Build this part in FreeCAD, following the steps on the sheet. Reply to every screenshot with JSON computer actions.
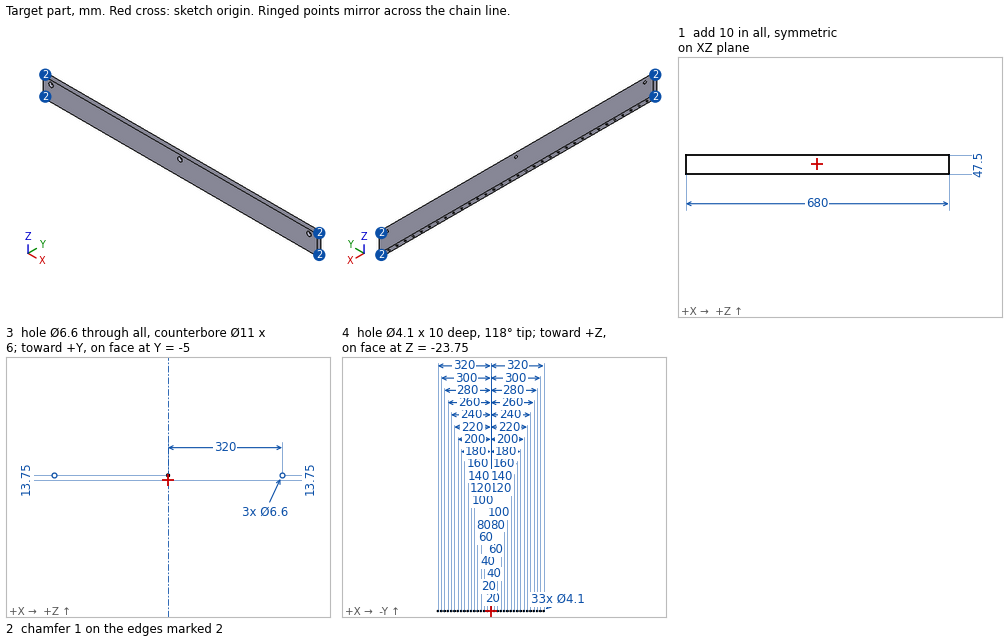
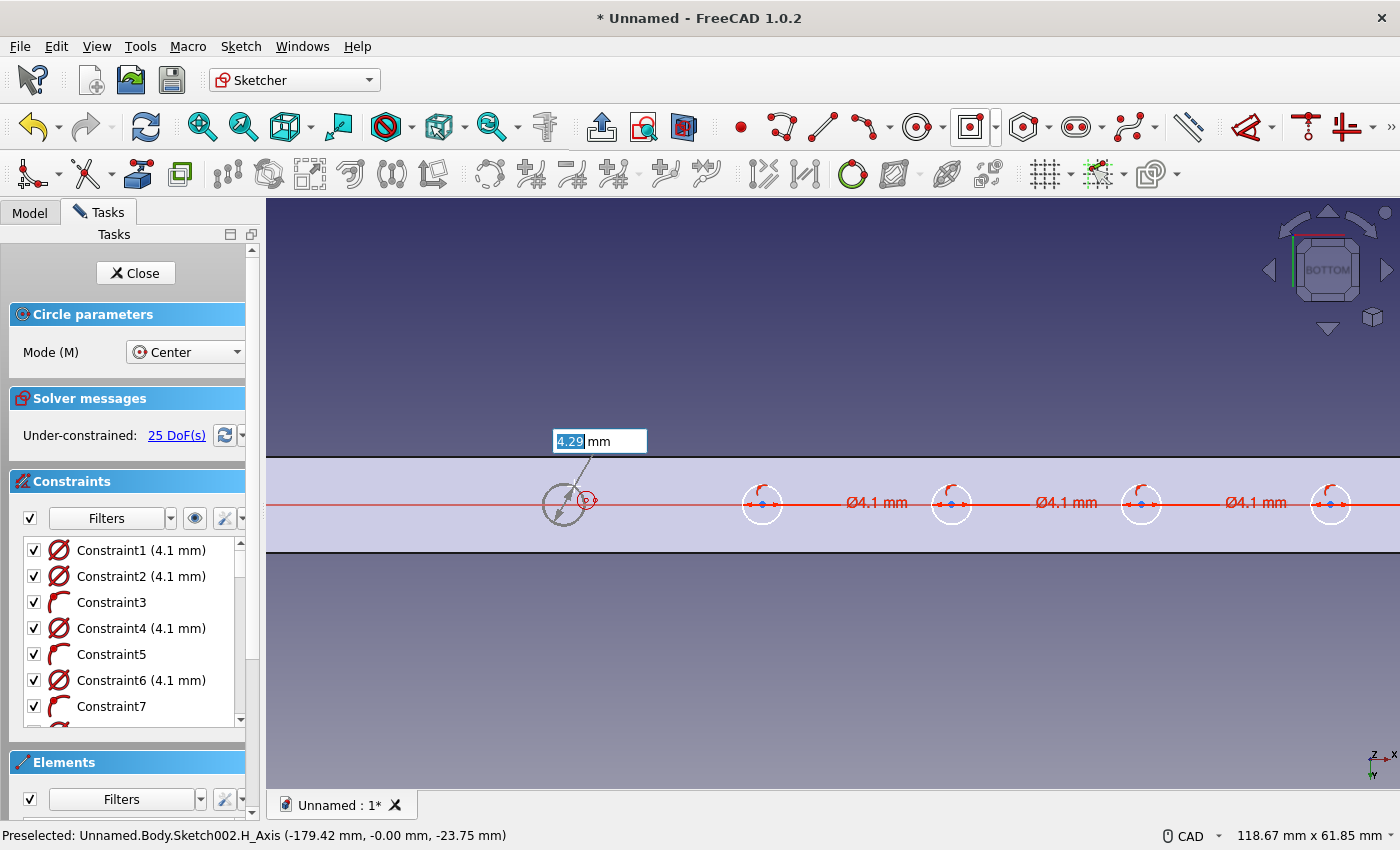
{"action": "type", "text": "4.1"}
{"action": "key", "text": "Return"}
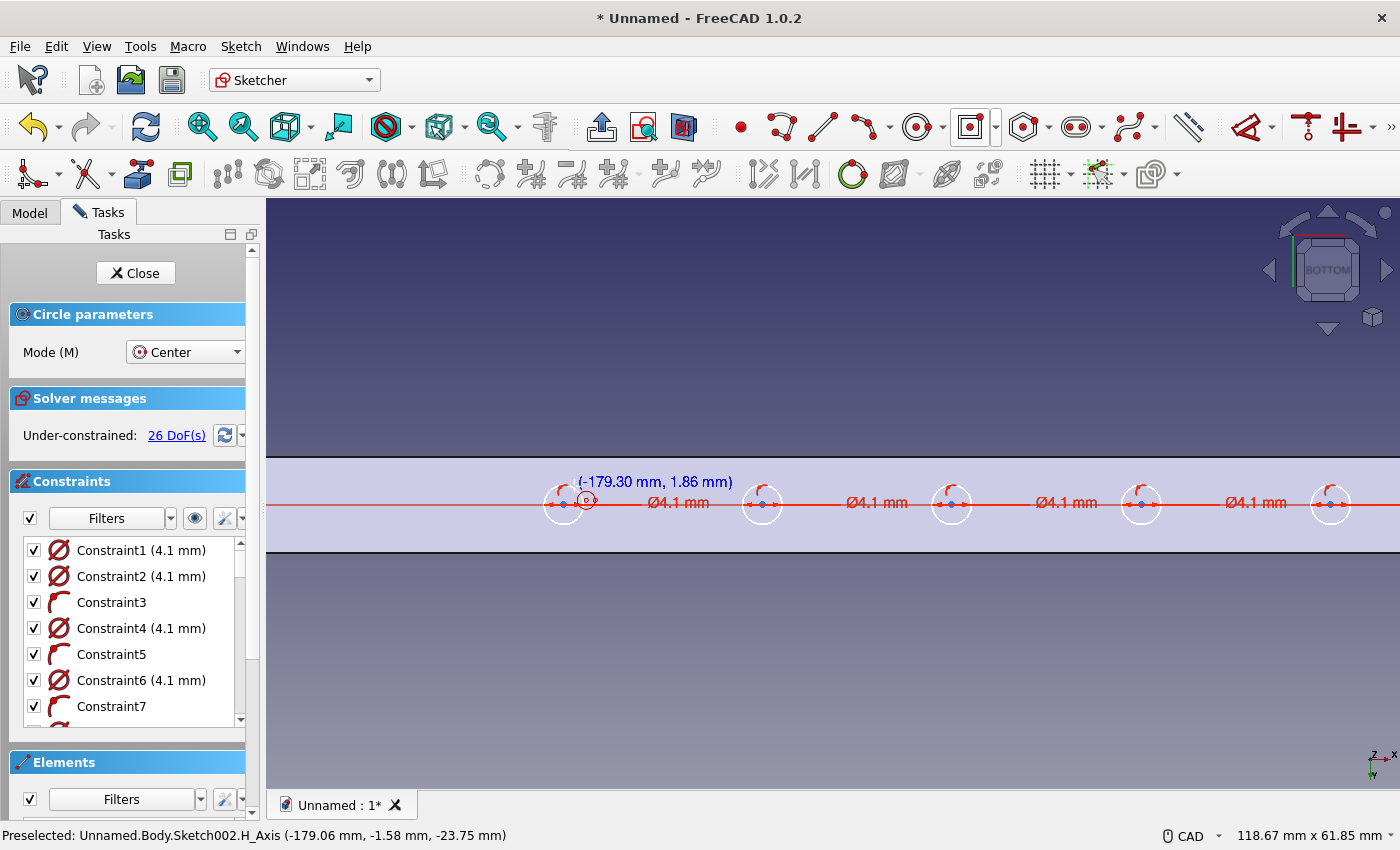
{"action": "scroll", "coordinate": [575, 492], "scroll_direction": "down", "scroll_amount": 11}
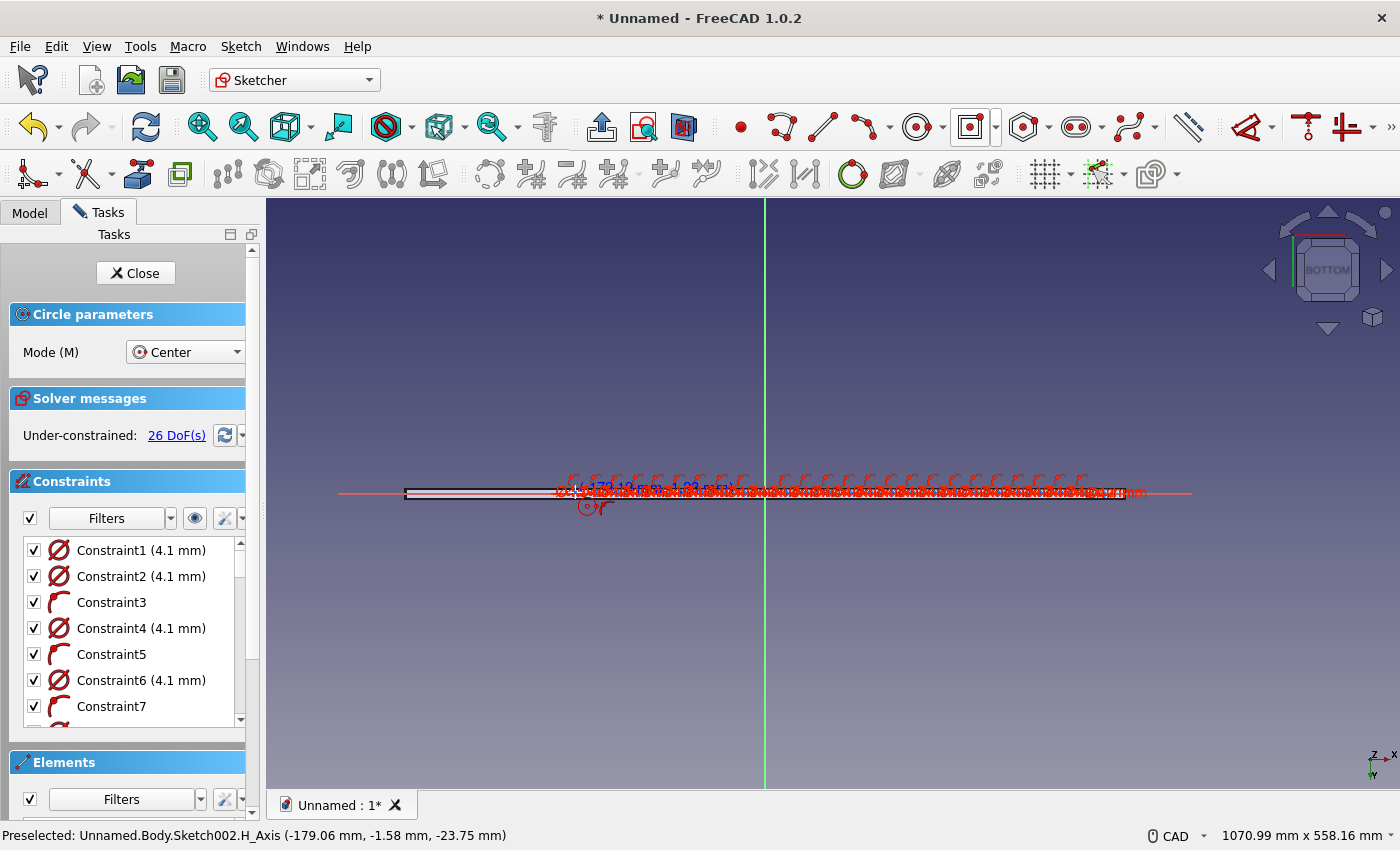
{"action": "left_click", "coordinate": [553, 494]}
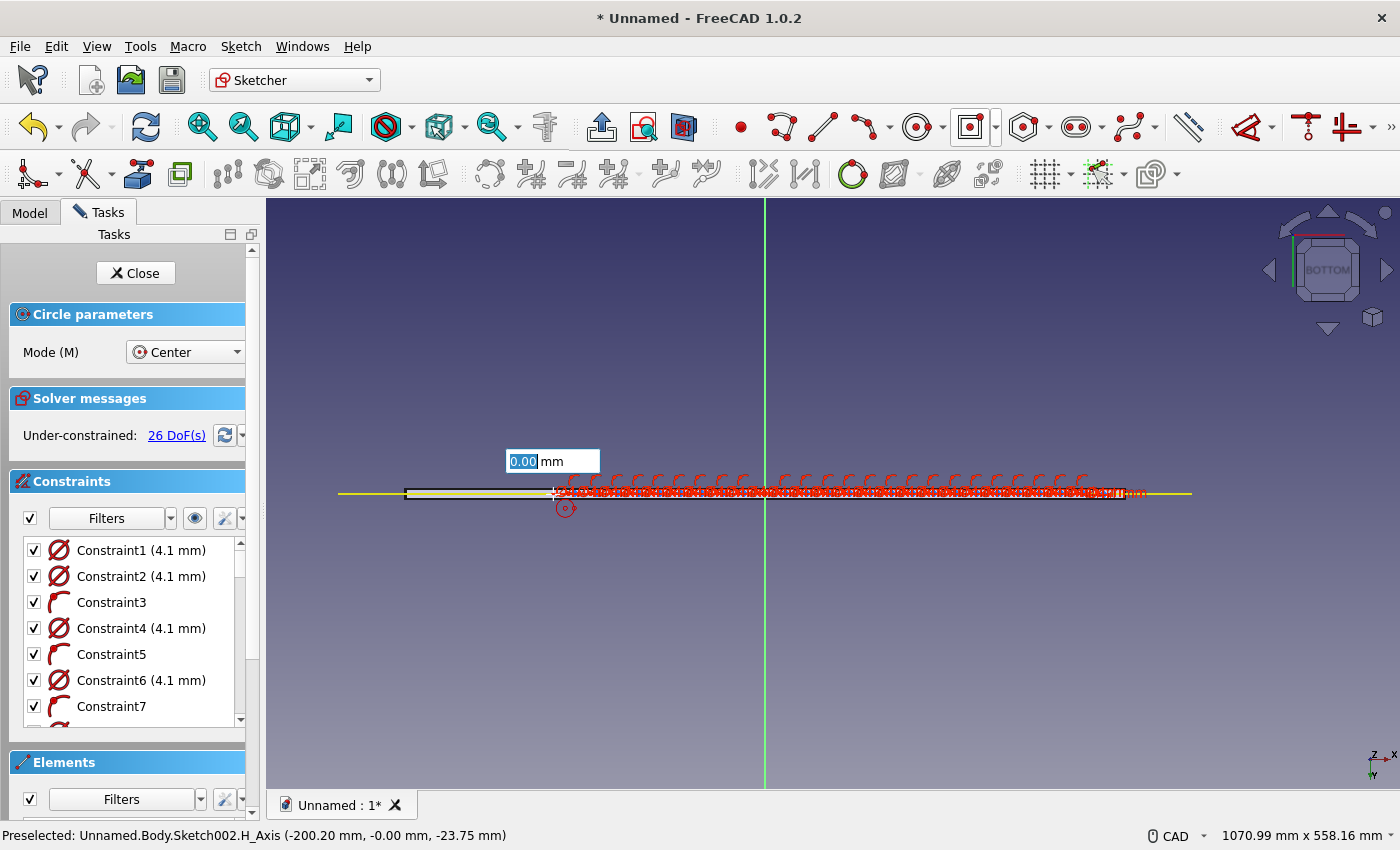
{"action": "scroll", "coordinate": [554, 492], "scroll_direction": "up", "scroll_amount": 11}
{"action": "mouse_move", "coordinate": [552, 486]}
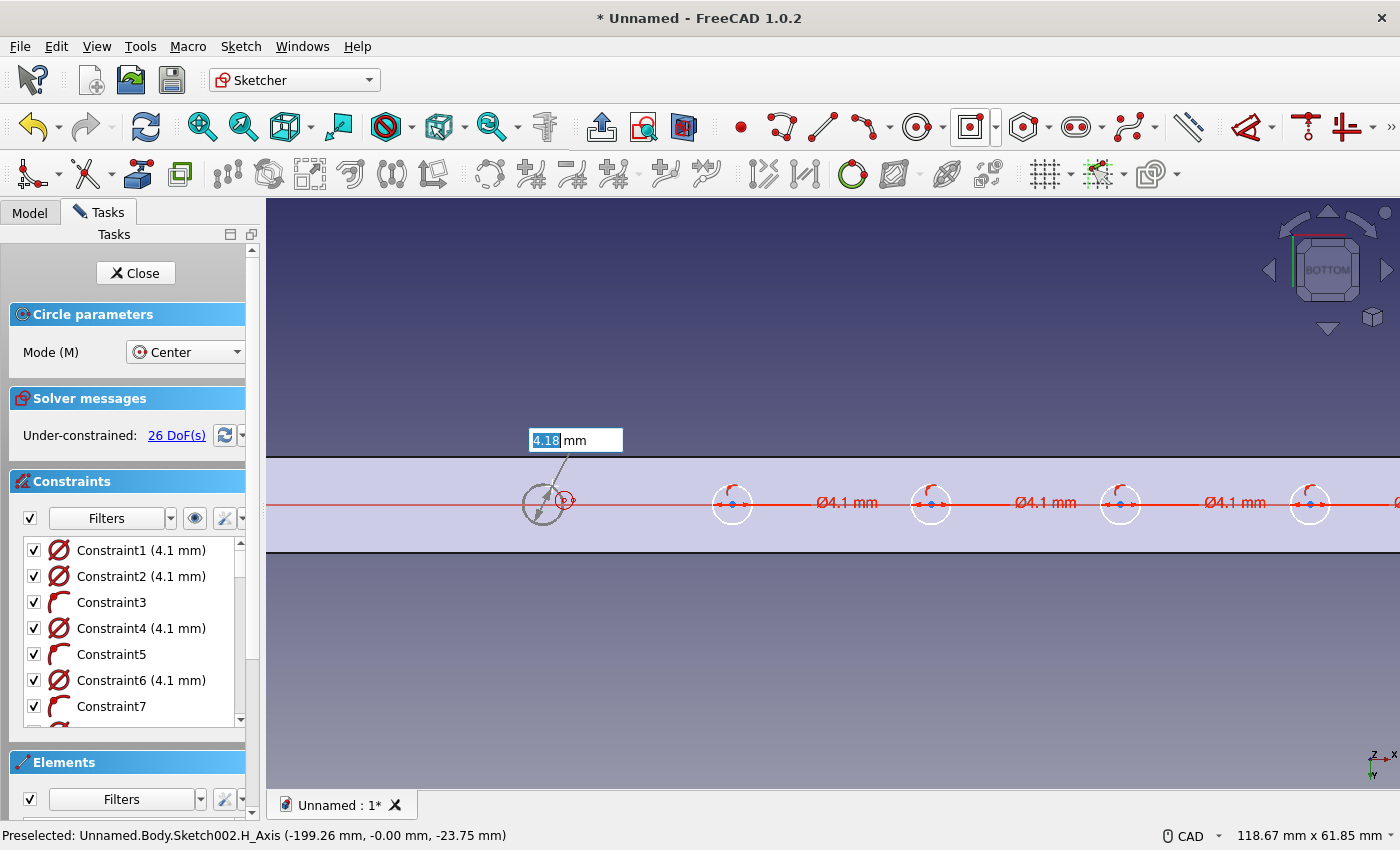
{"action": "type", "text": "4.1"}
{"action": "key", "text": "Return"}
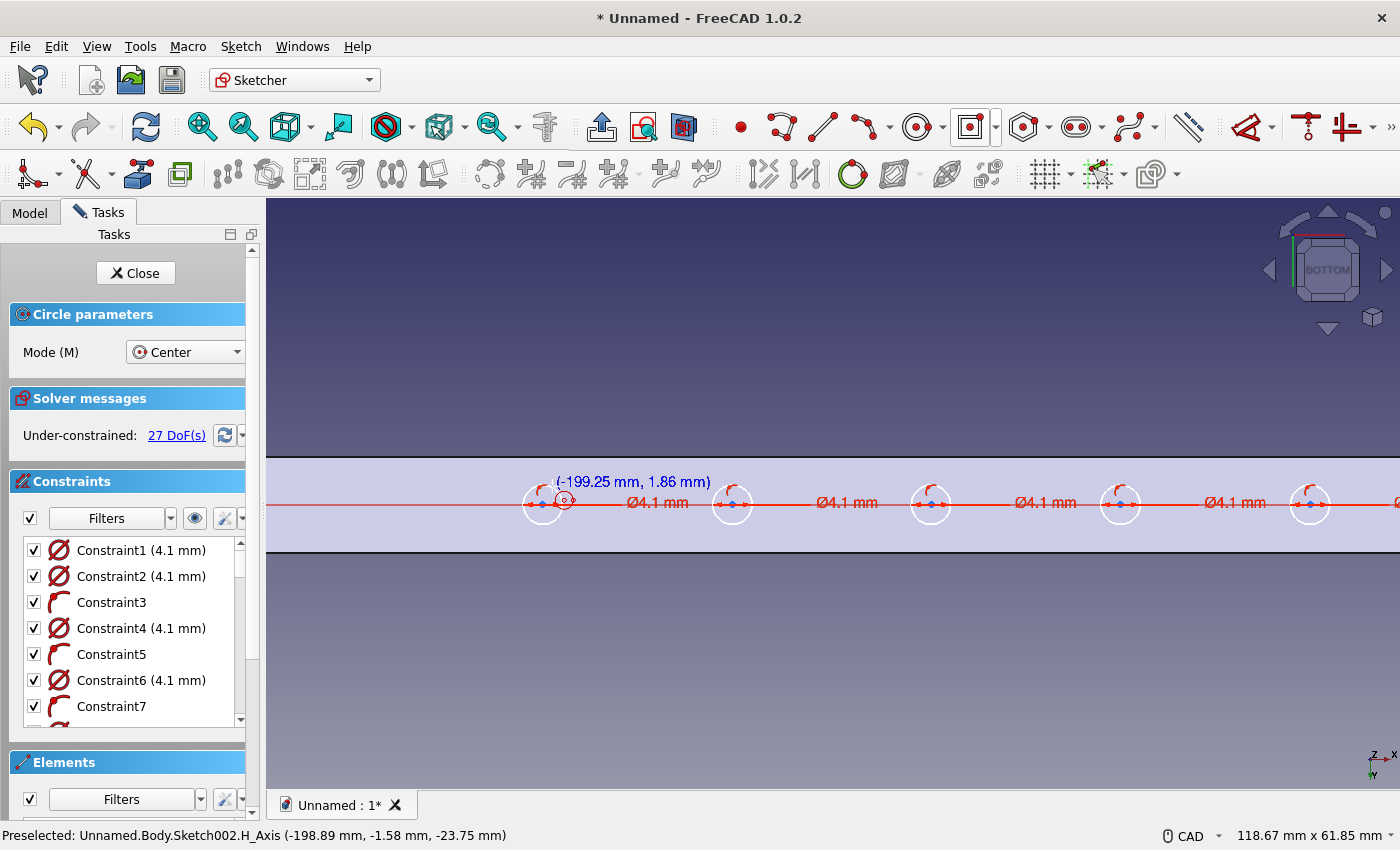
{"action": "scroll", "coordinate": [554, 492], "scroll_direction": "down", "scroll_amount": 11}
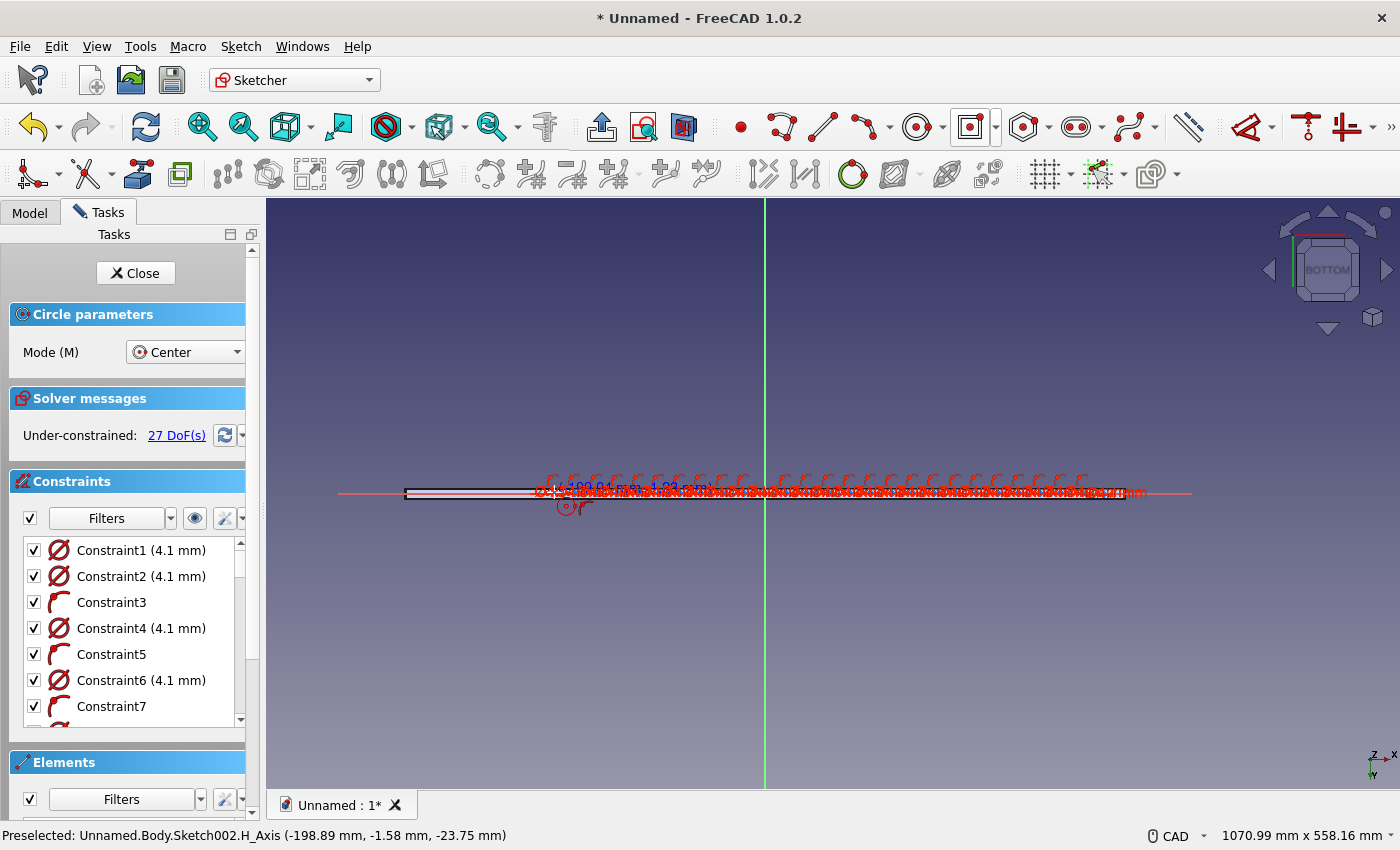
{"action": "left_click", "coordinate": [532, 494]}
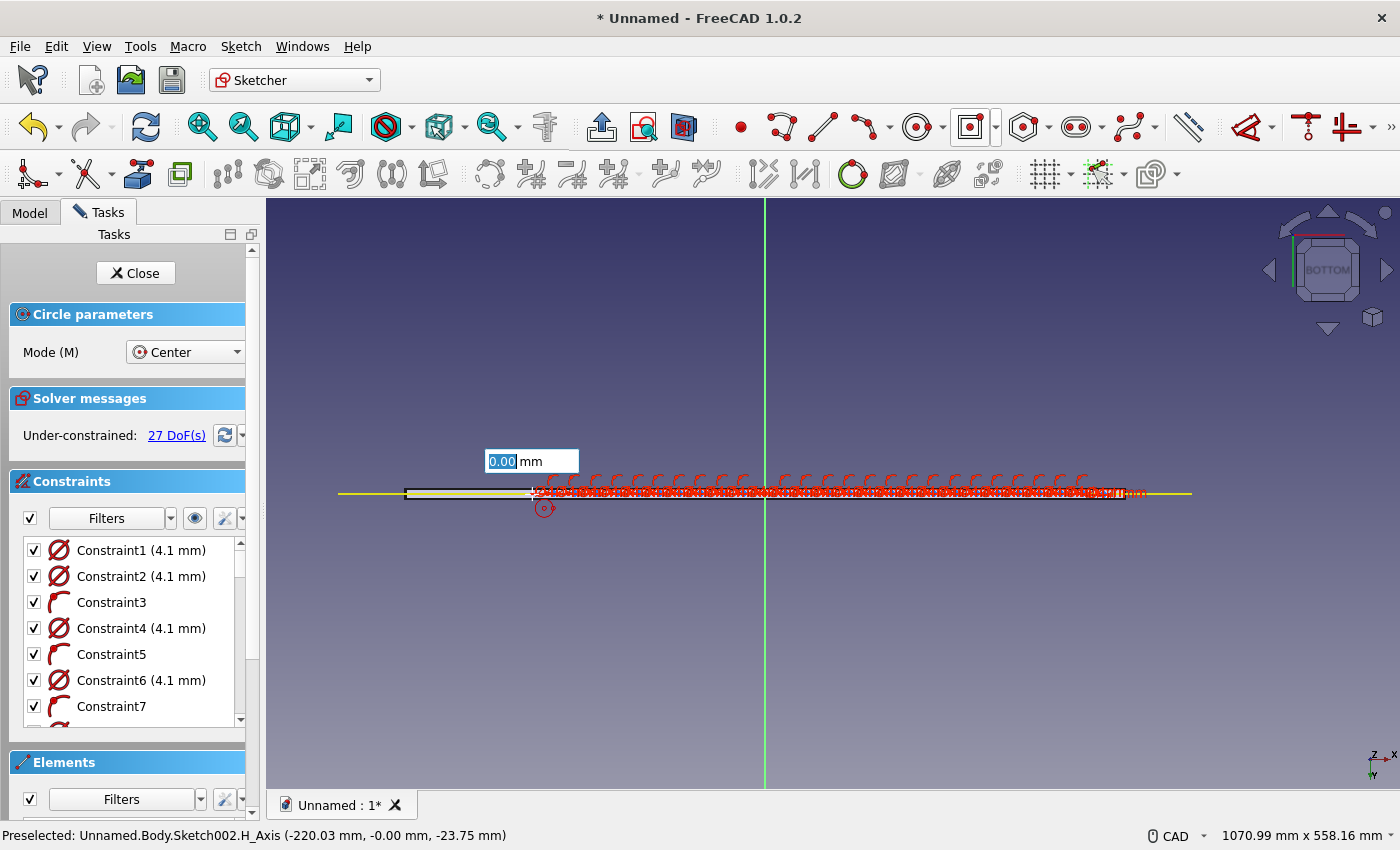
{"action": "scroll", "coordinate": [533, 492], "scroll_direction": "up", "scroll_amount": 11}
{"action": "mouse_move", "coordinate": [529, 486]}